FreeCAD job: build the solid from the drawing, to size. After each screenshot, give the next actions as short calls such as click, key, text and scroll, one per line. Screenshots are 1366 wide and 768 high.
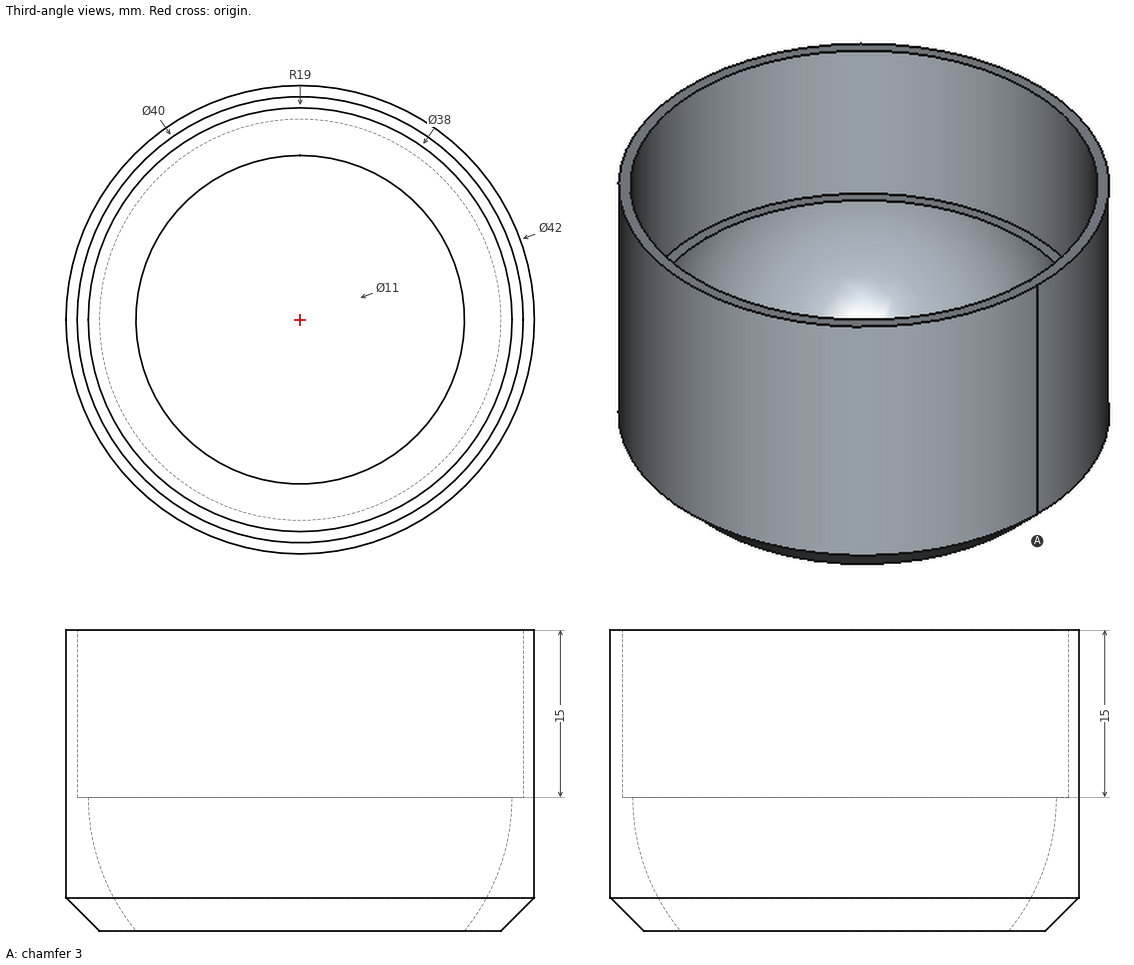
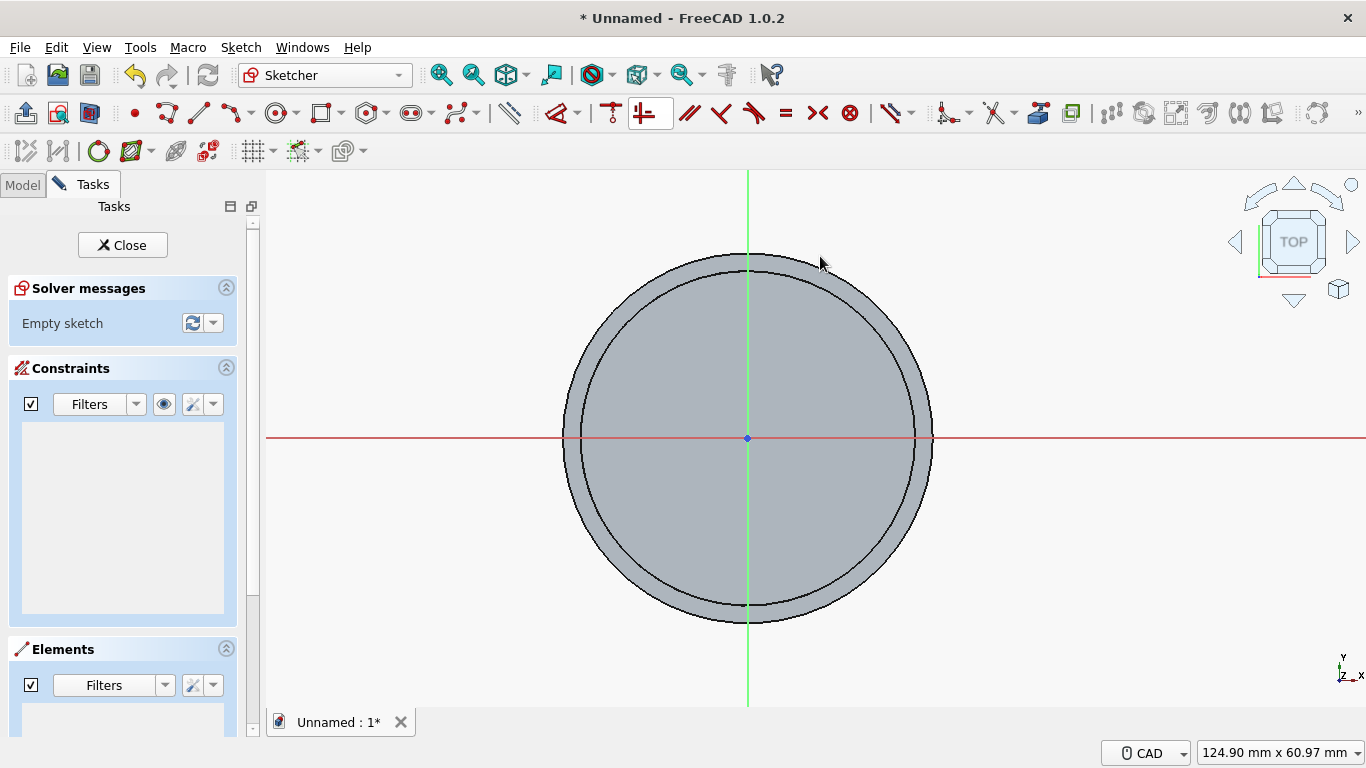
click(276, 114)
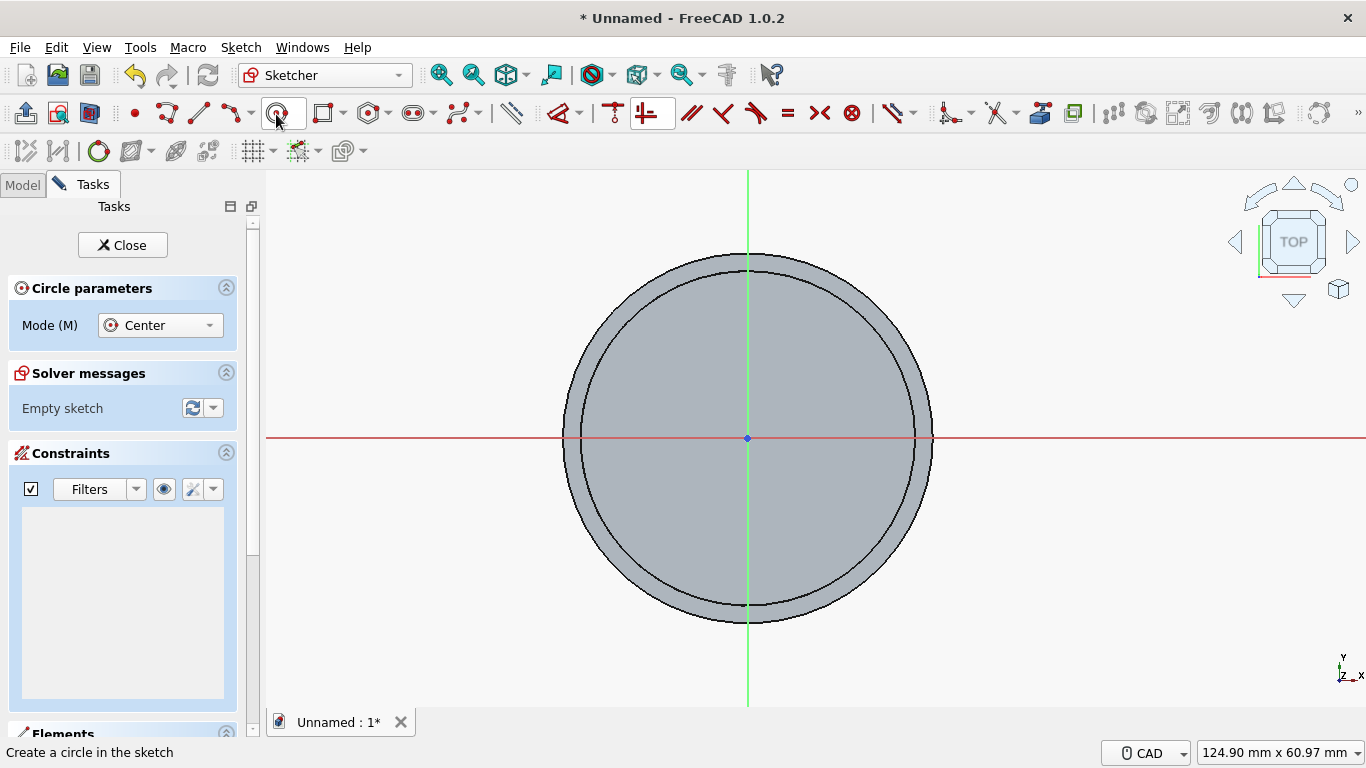
click(748, 438)
move(872, 314)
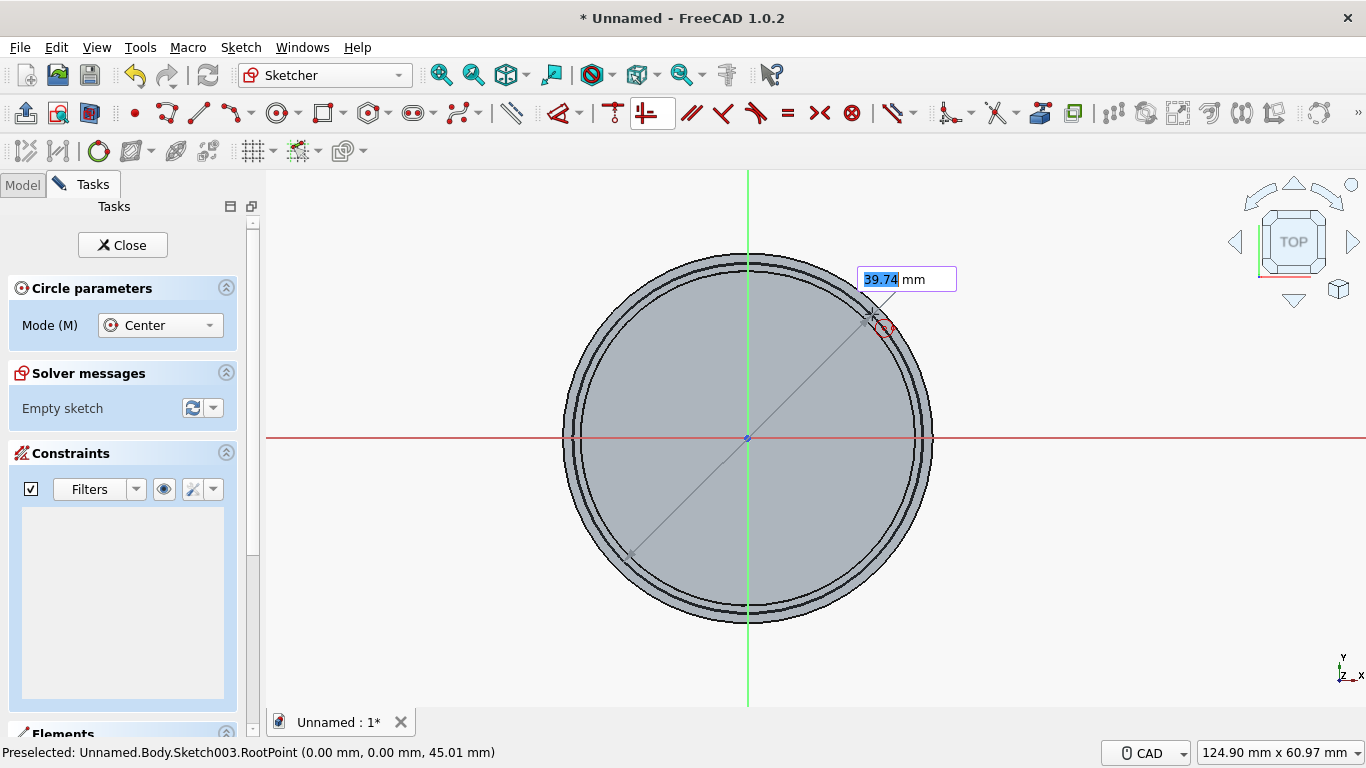
text(40)
key(Return)
key(Escape)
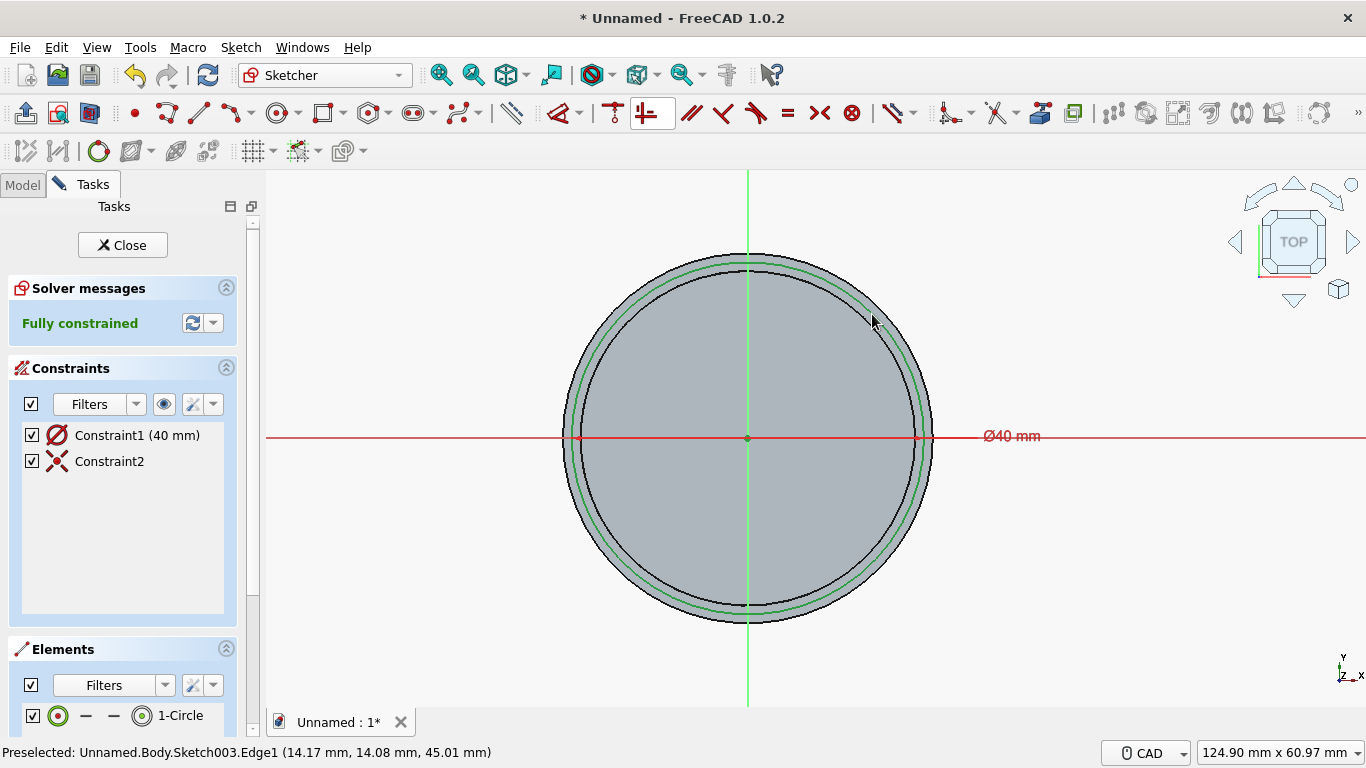
click(123, 245)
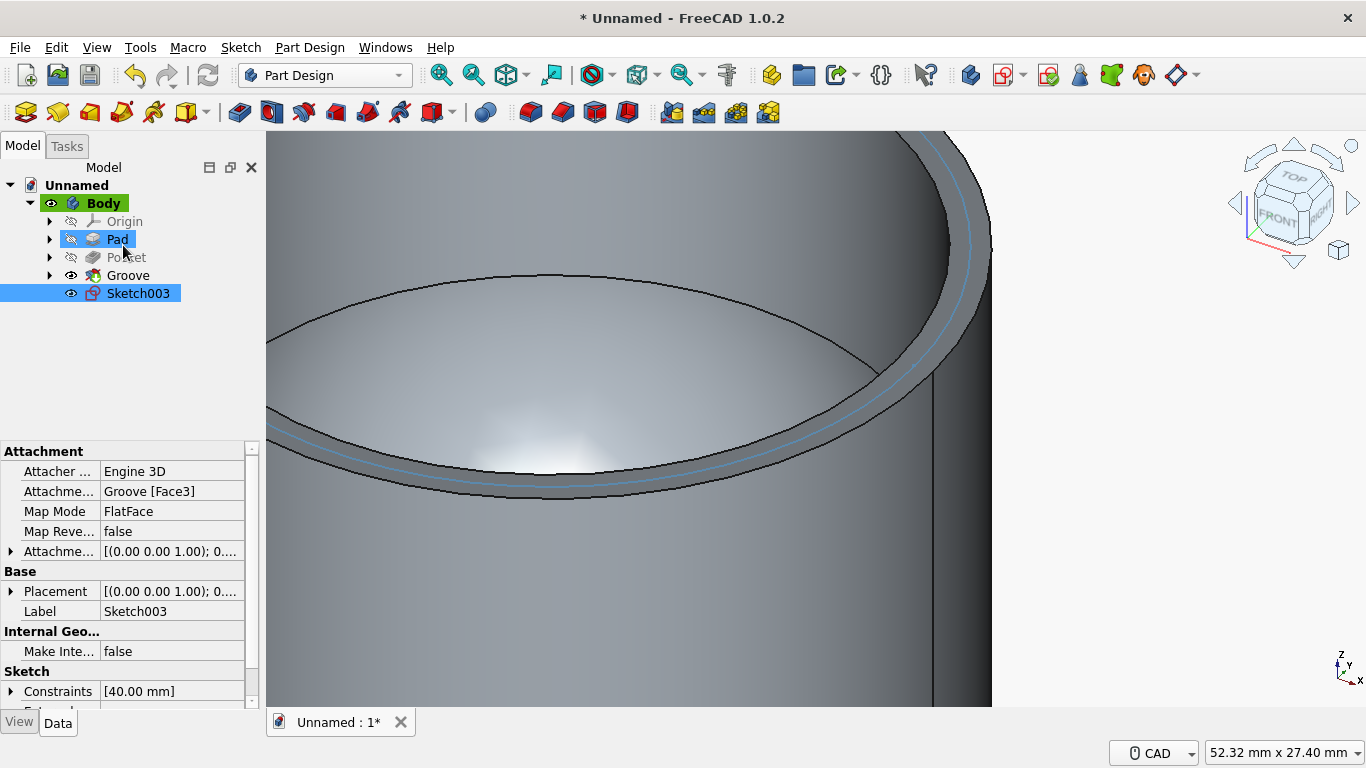
click(240, 112)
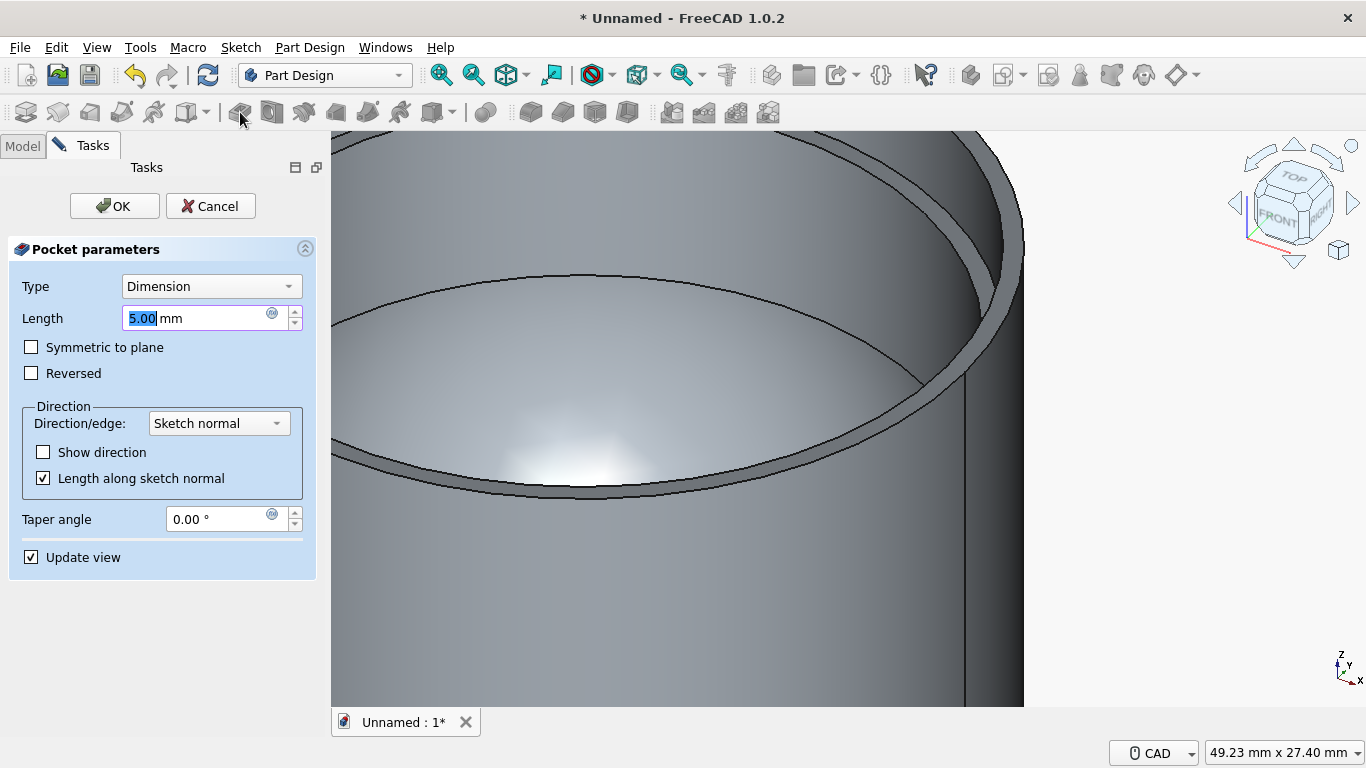
text(15)
key(Tab)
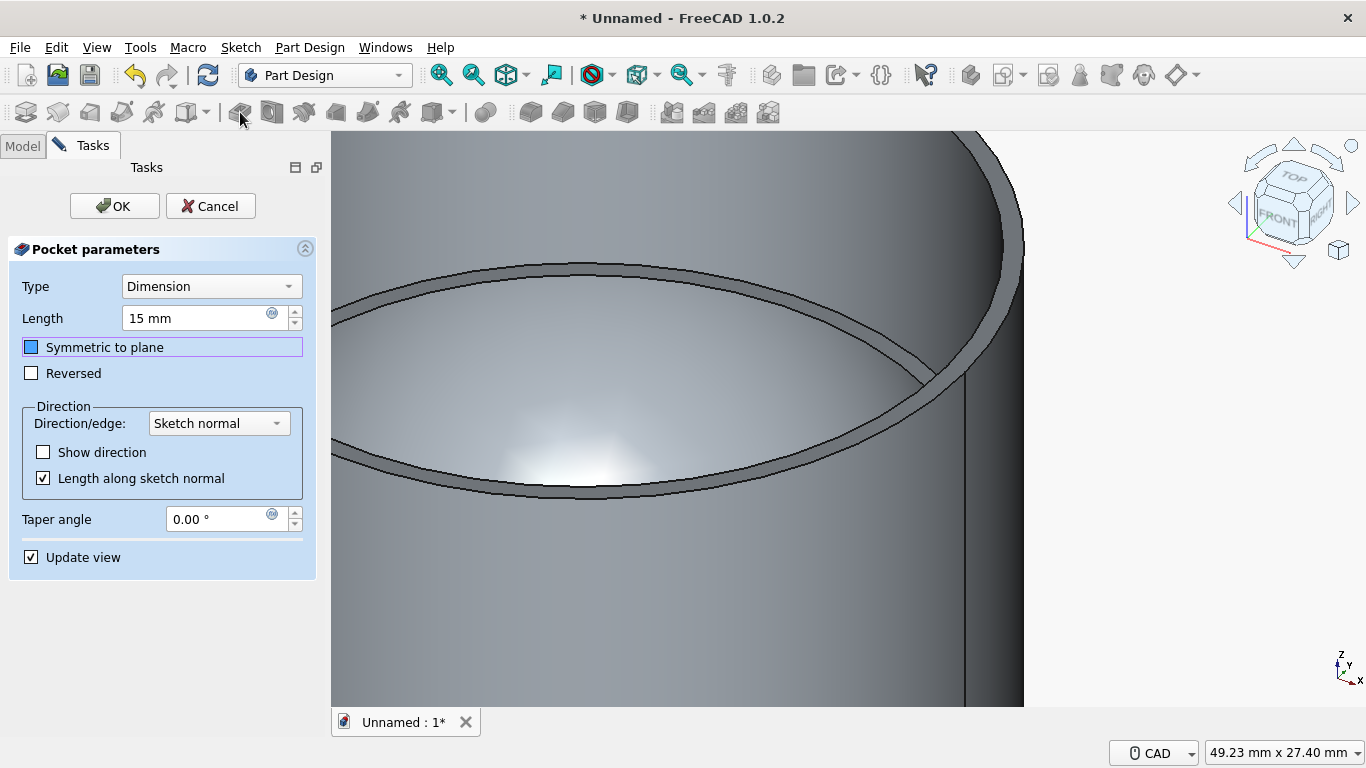
click(115, 206)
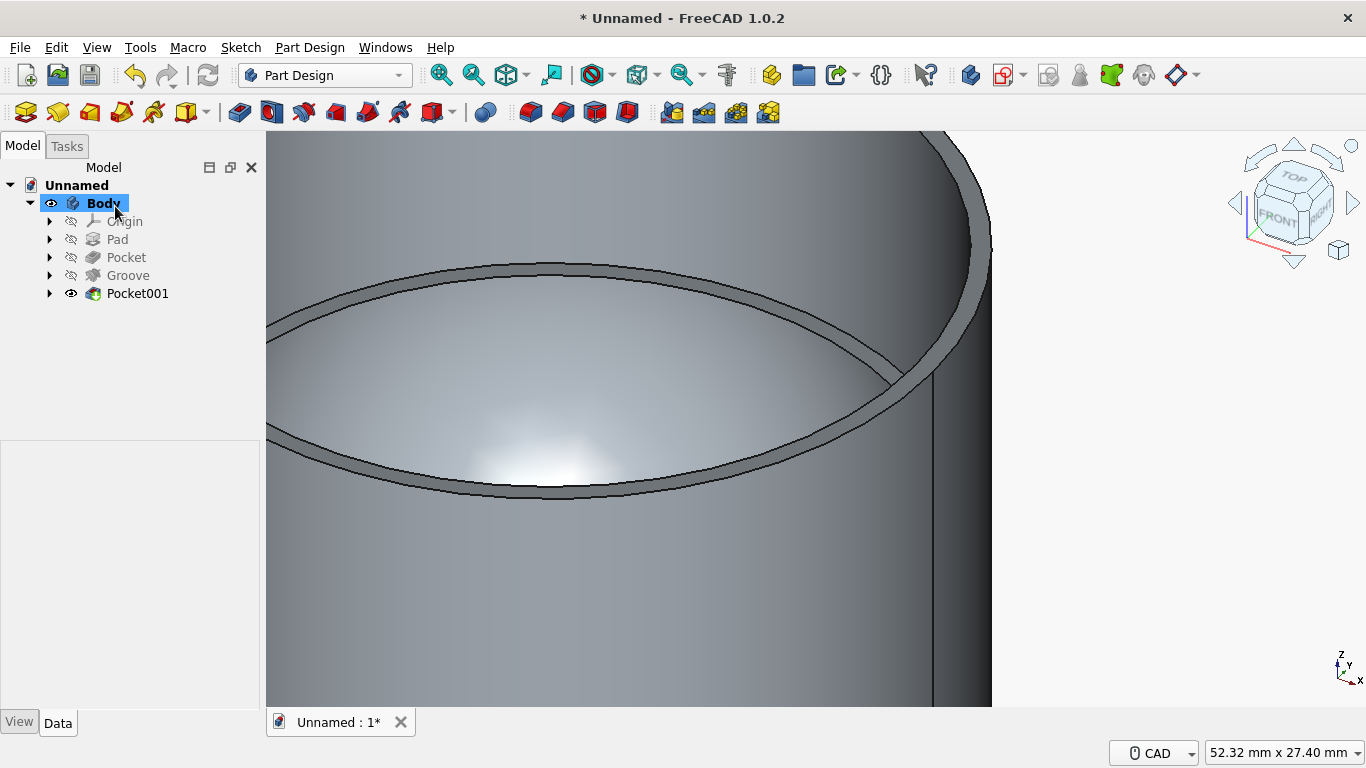
click(442, 76)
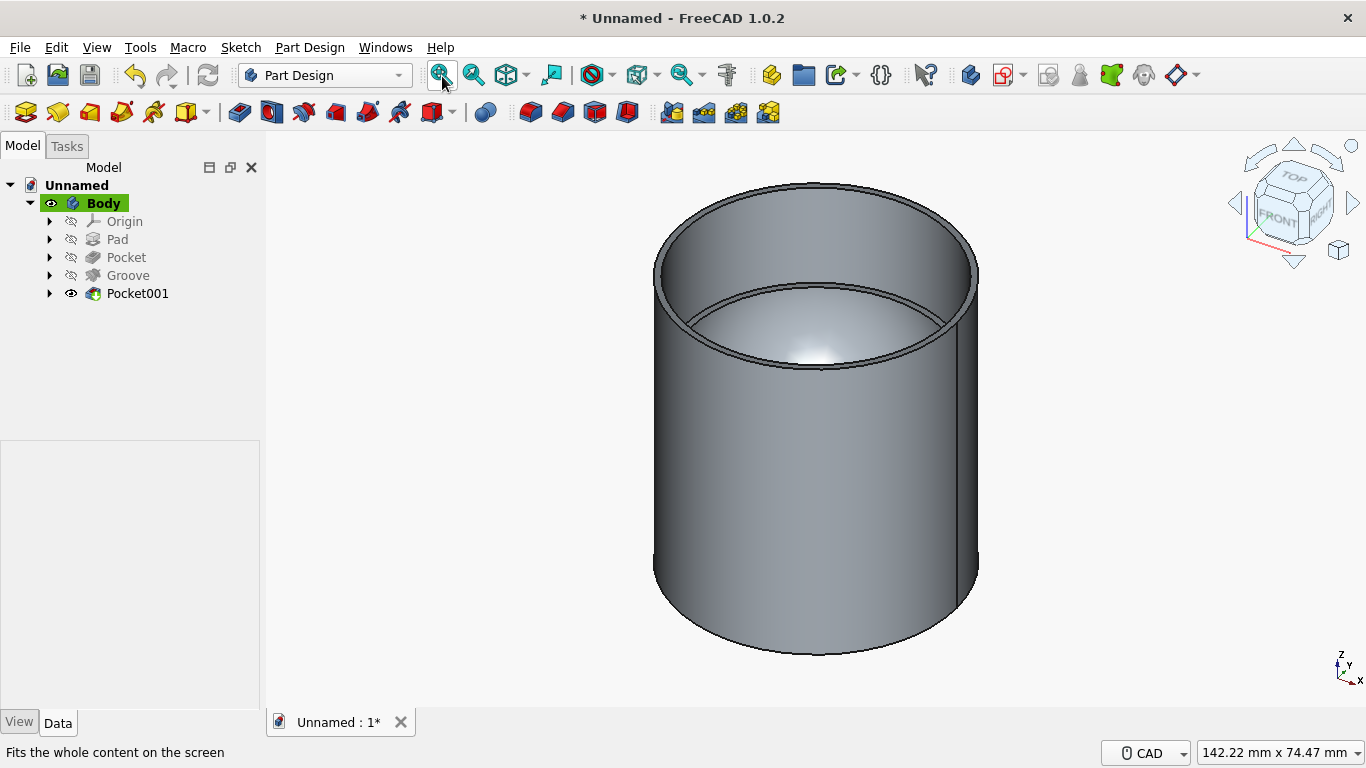
key(5)